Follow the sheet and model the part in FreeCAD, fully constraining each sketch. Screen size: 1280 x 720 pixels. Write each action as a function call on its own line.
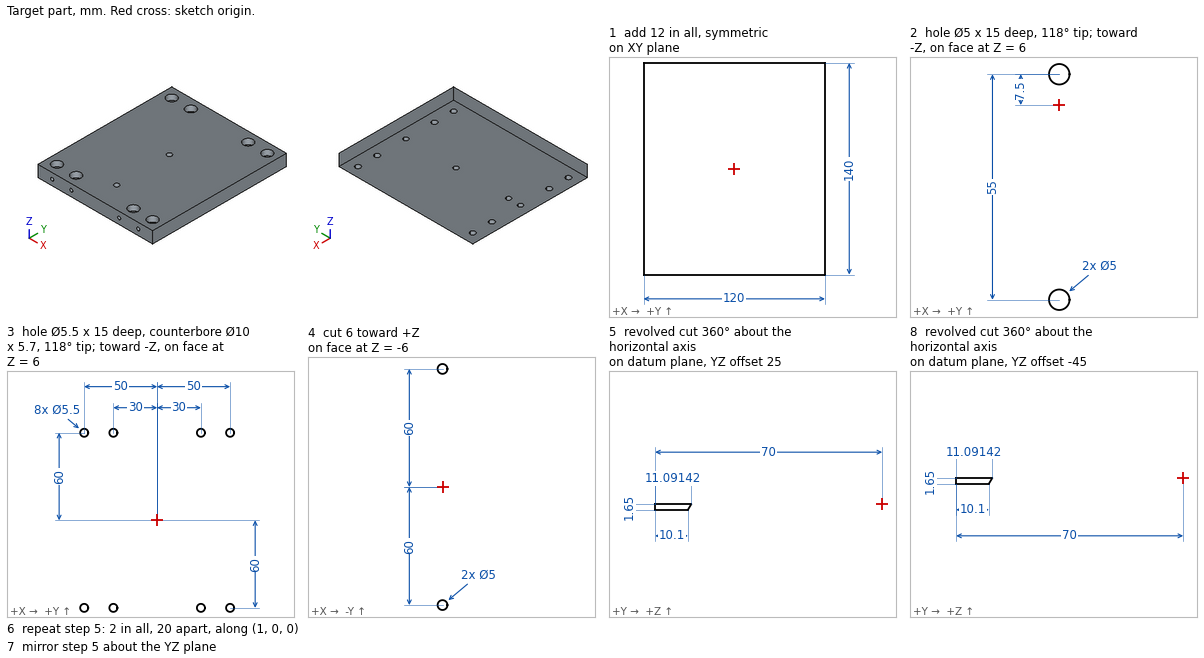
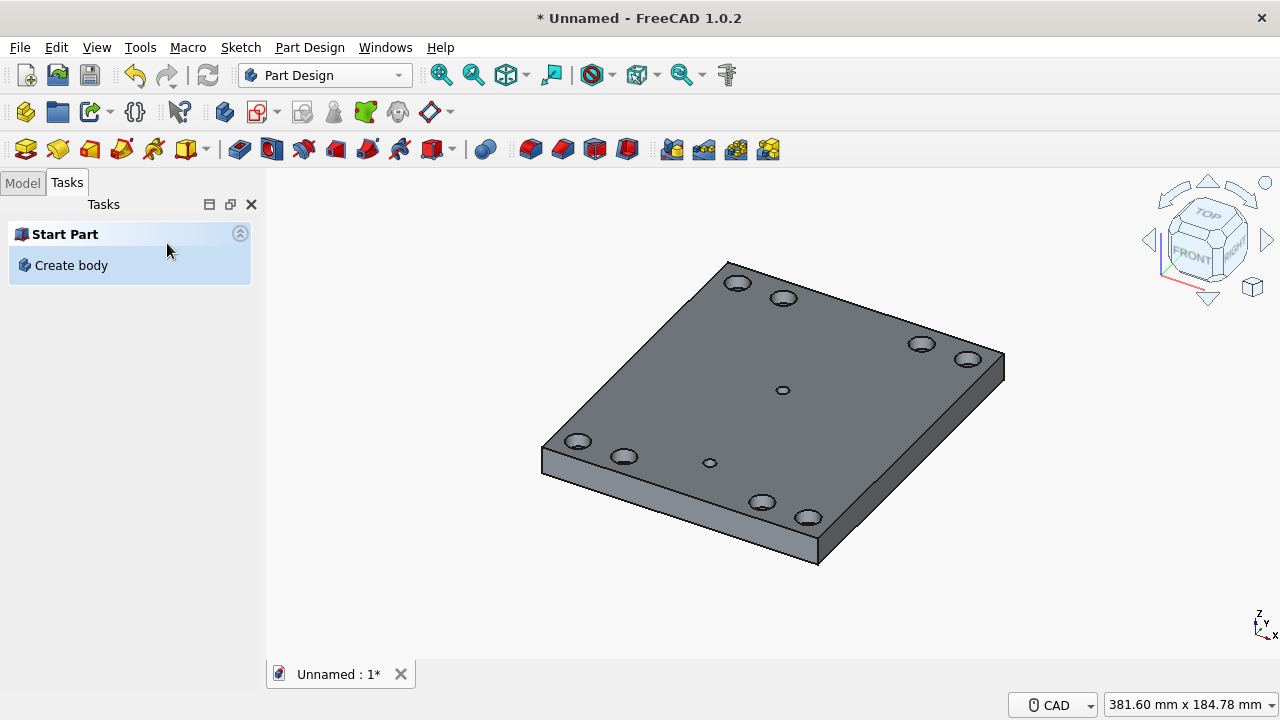
key(5)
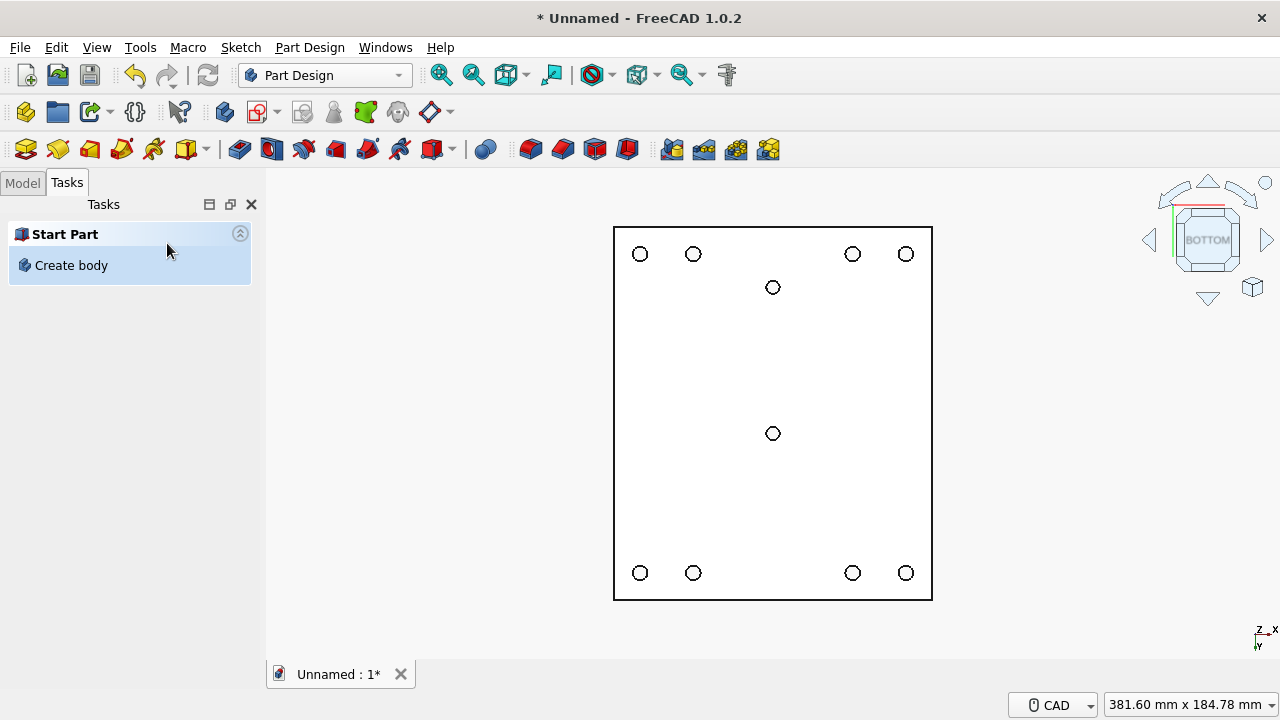
click(773, 519)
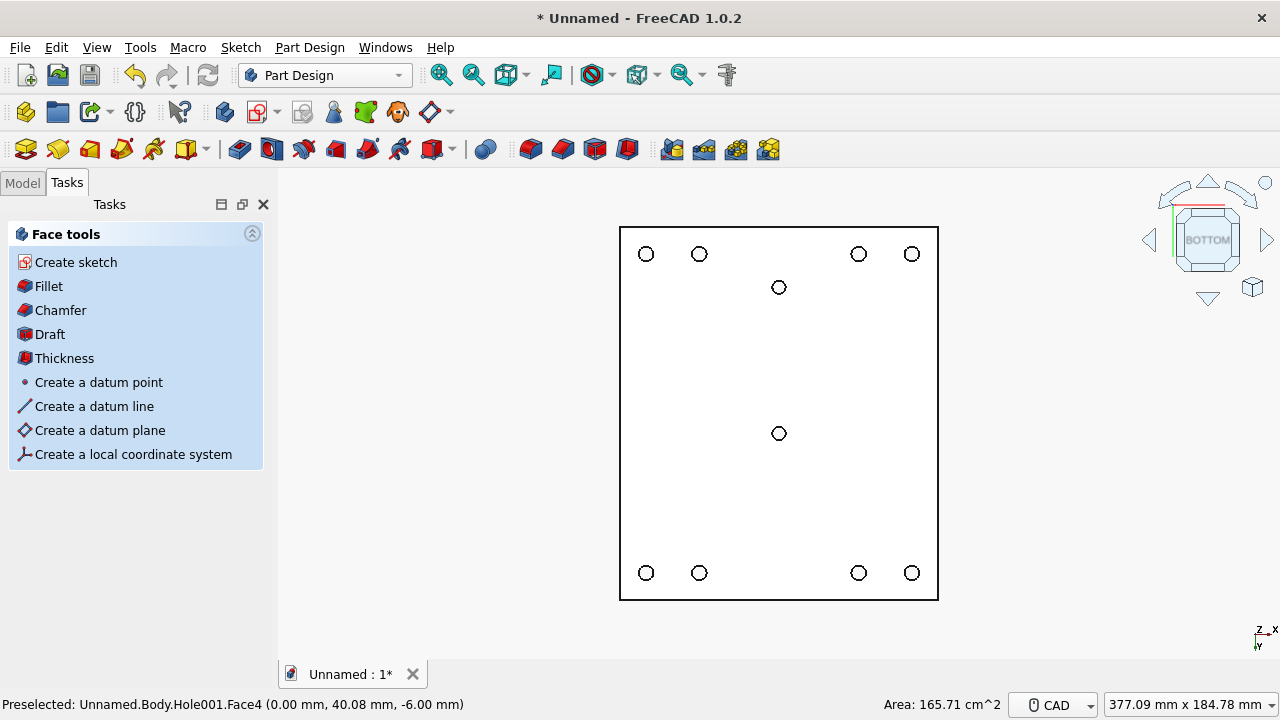
click(258, 112)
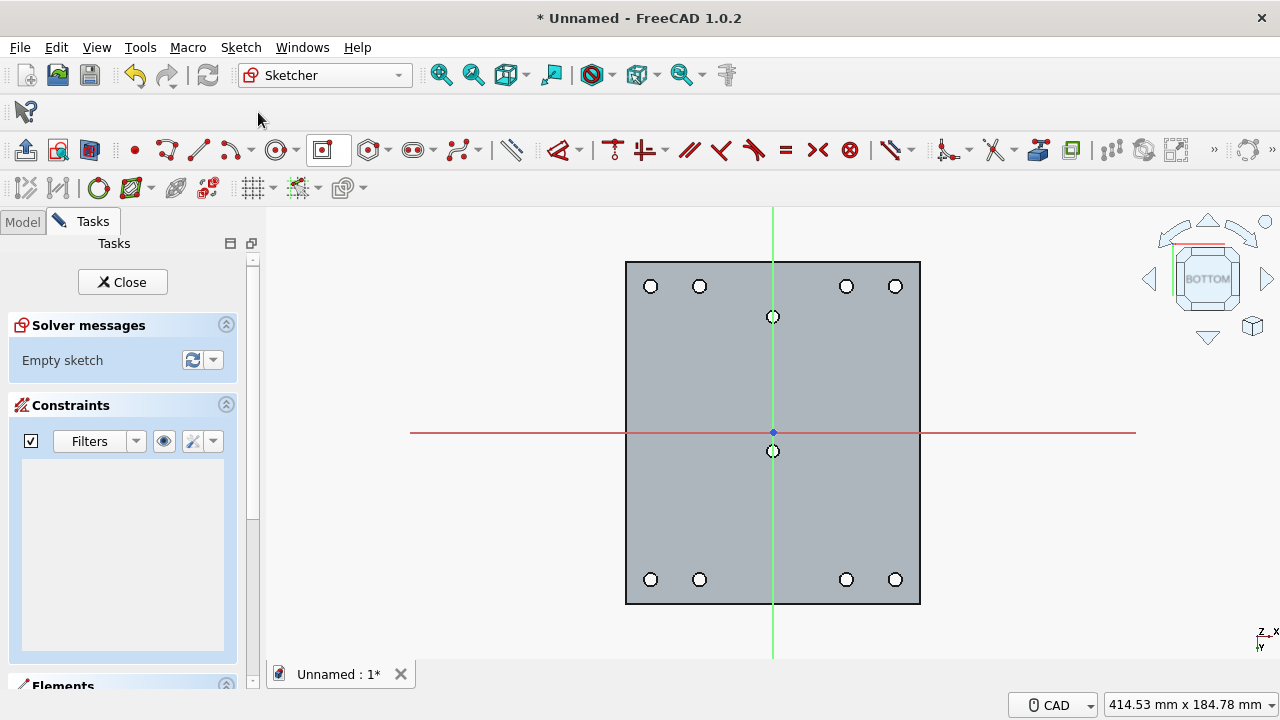
key(g)
key(c)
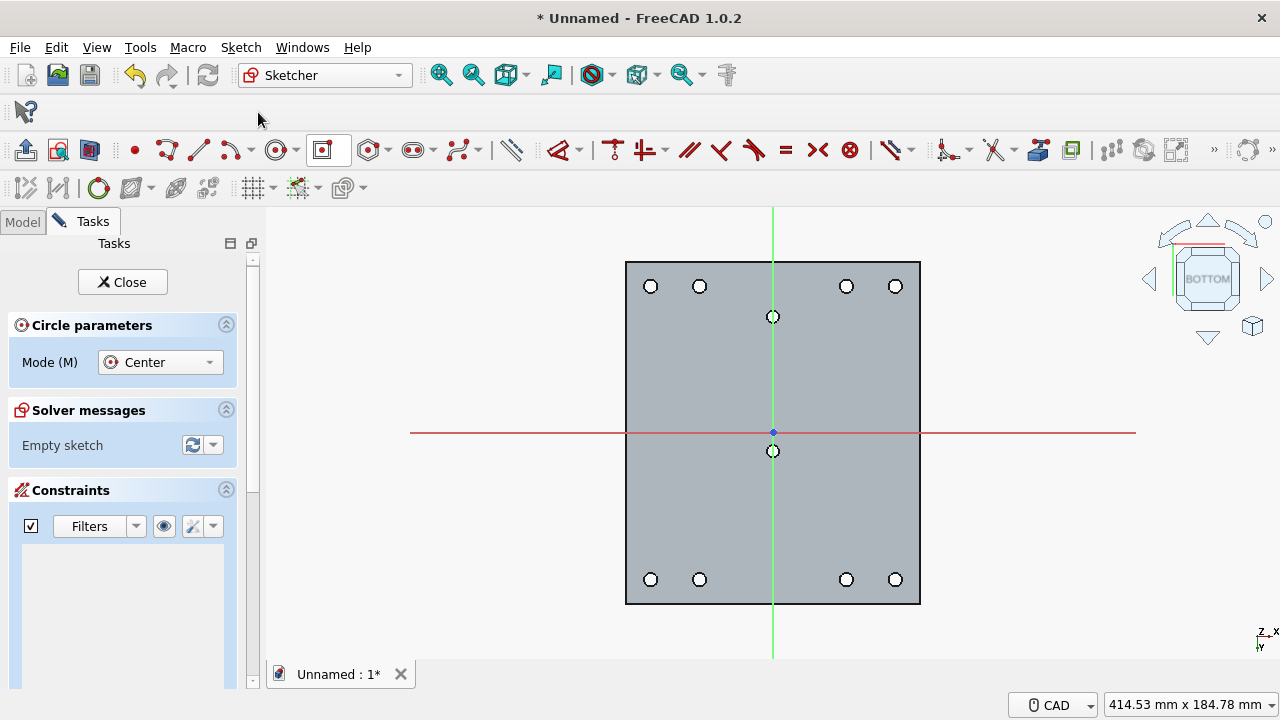
scroll(773, 580, up, 7)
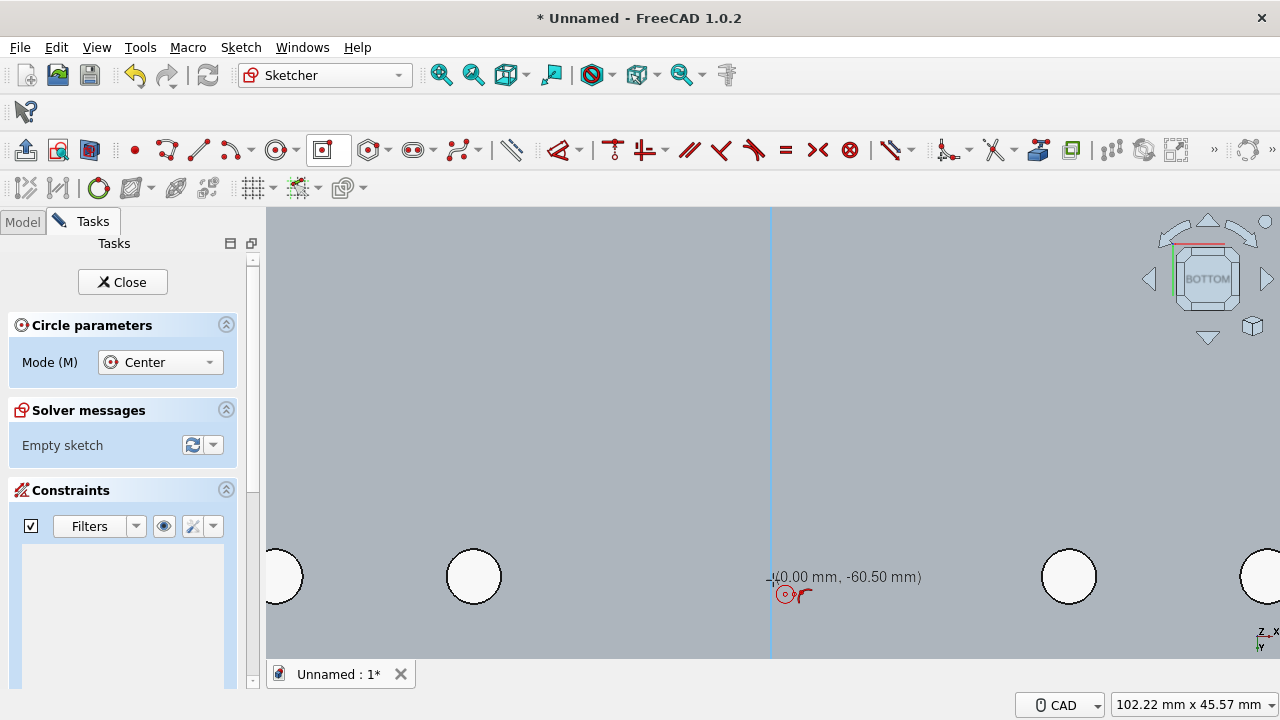
scroll(683, 581, down, 7)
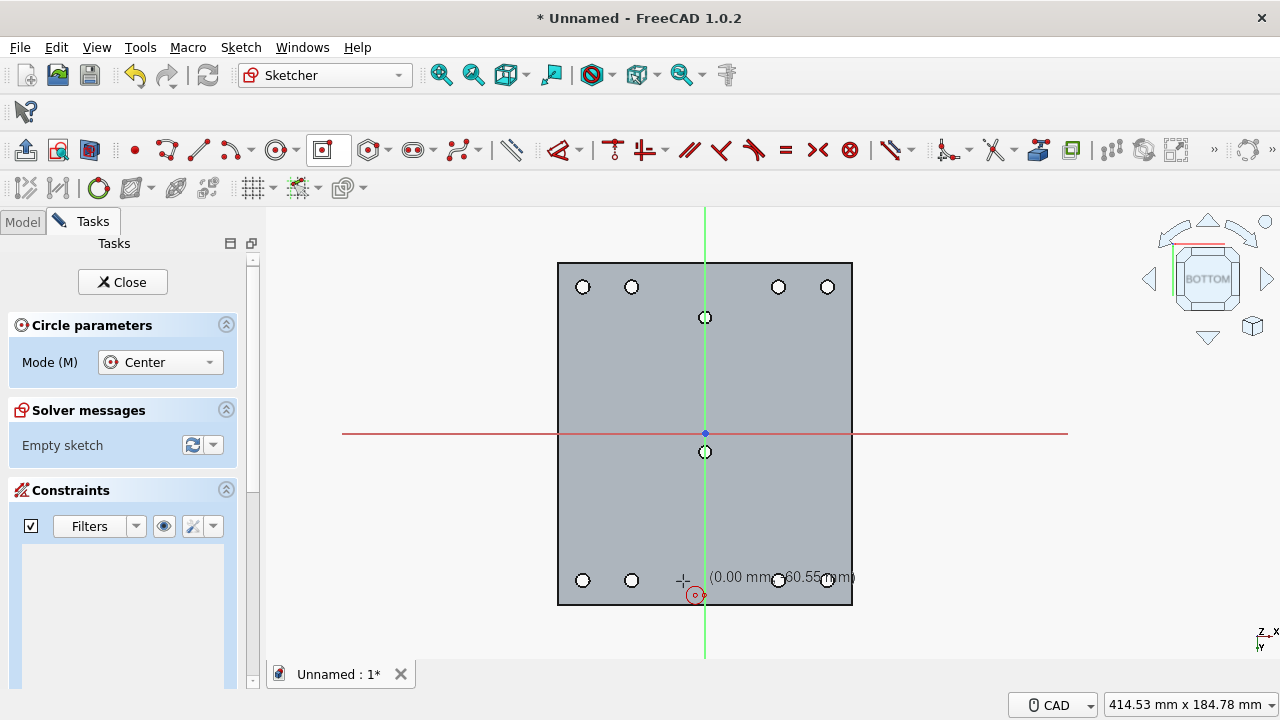
click(705, 581)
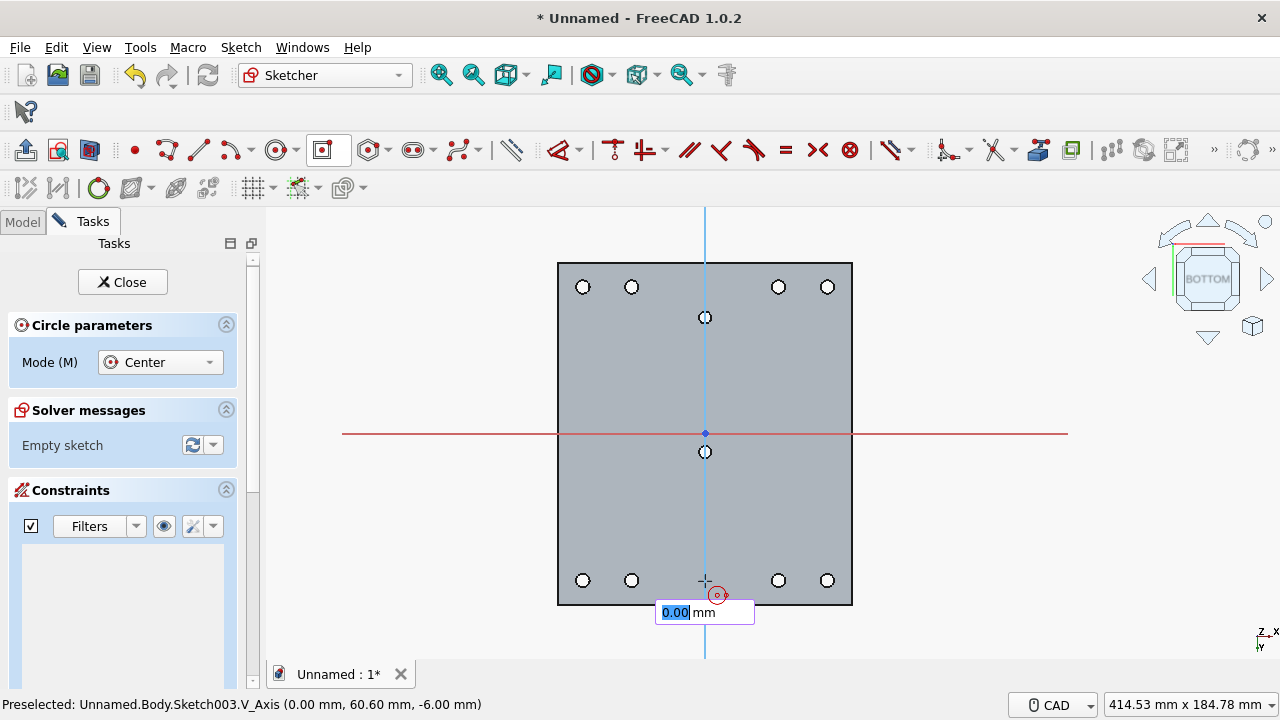
scroll(711, 578, up, 6)
move(710, 578)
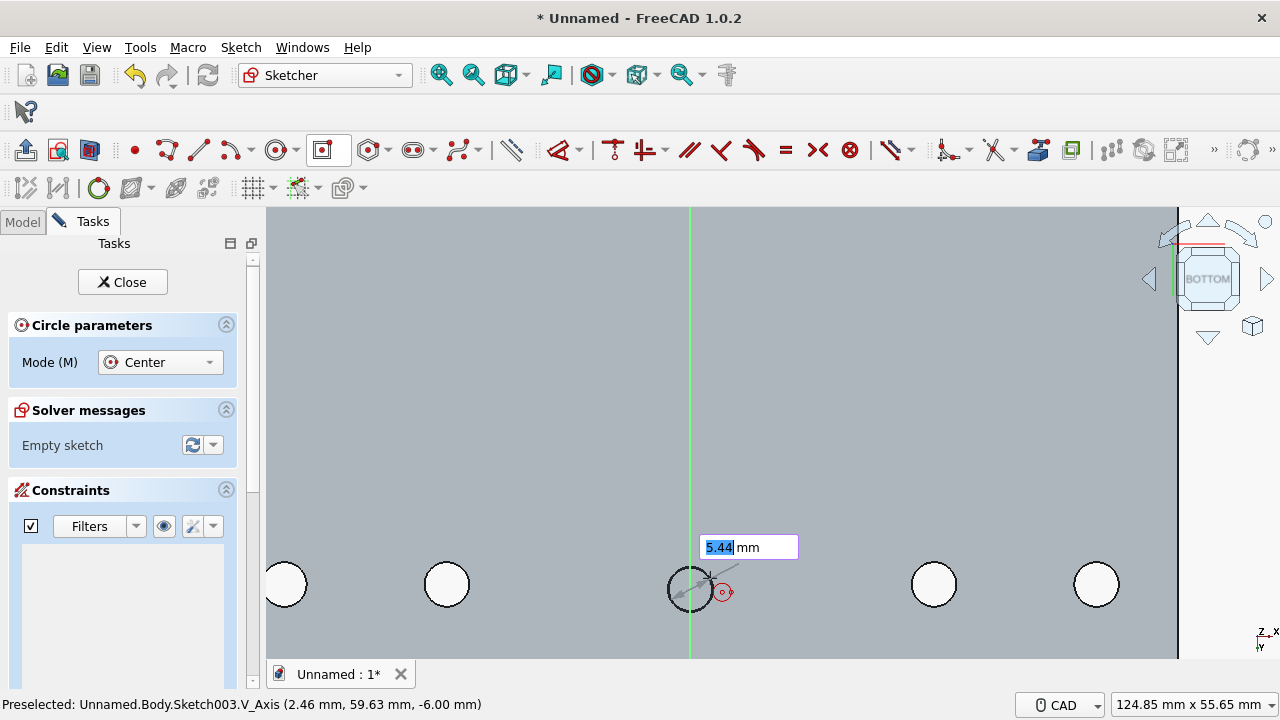
text(5)
key(Return)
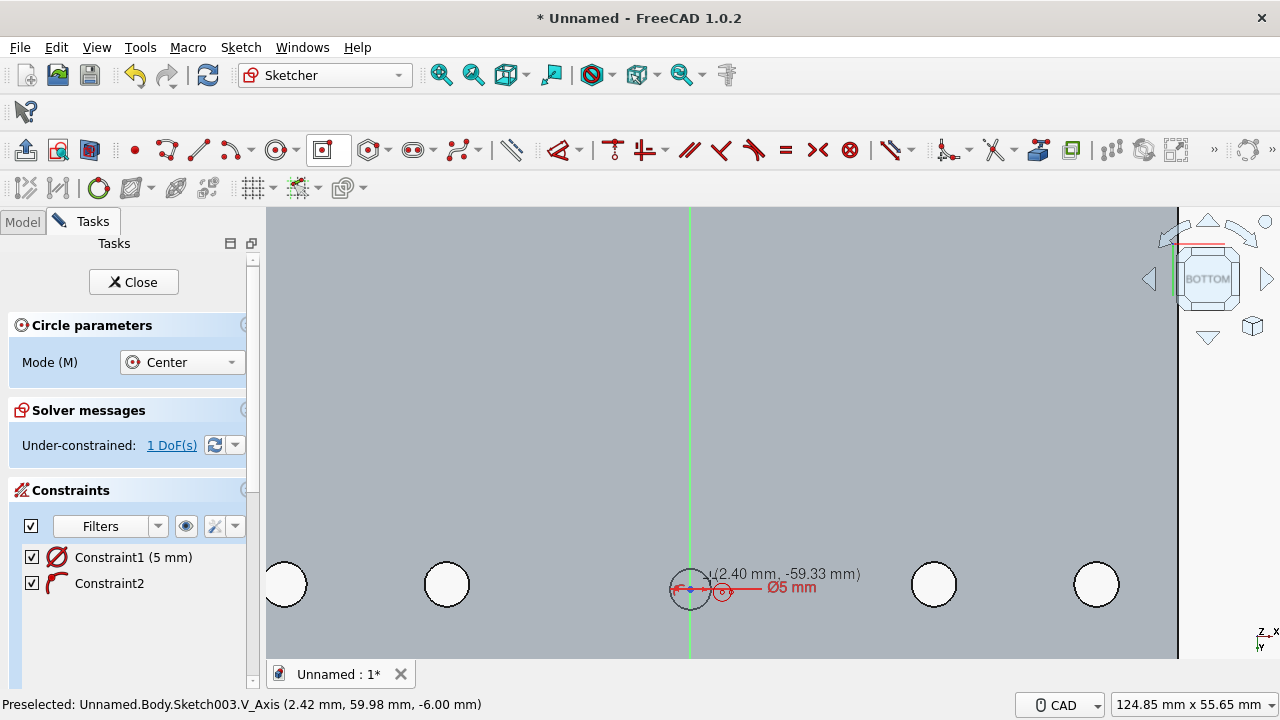
scroll(711, 578, down, 6)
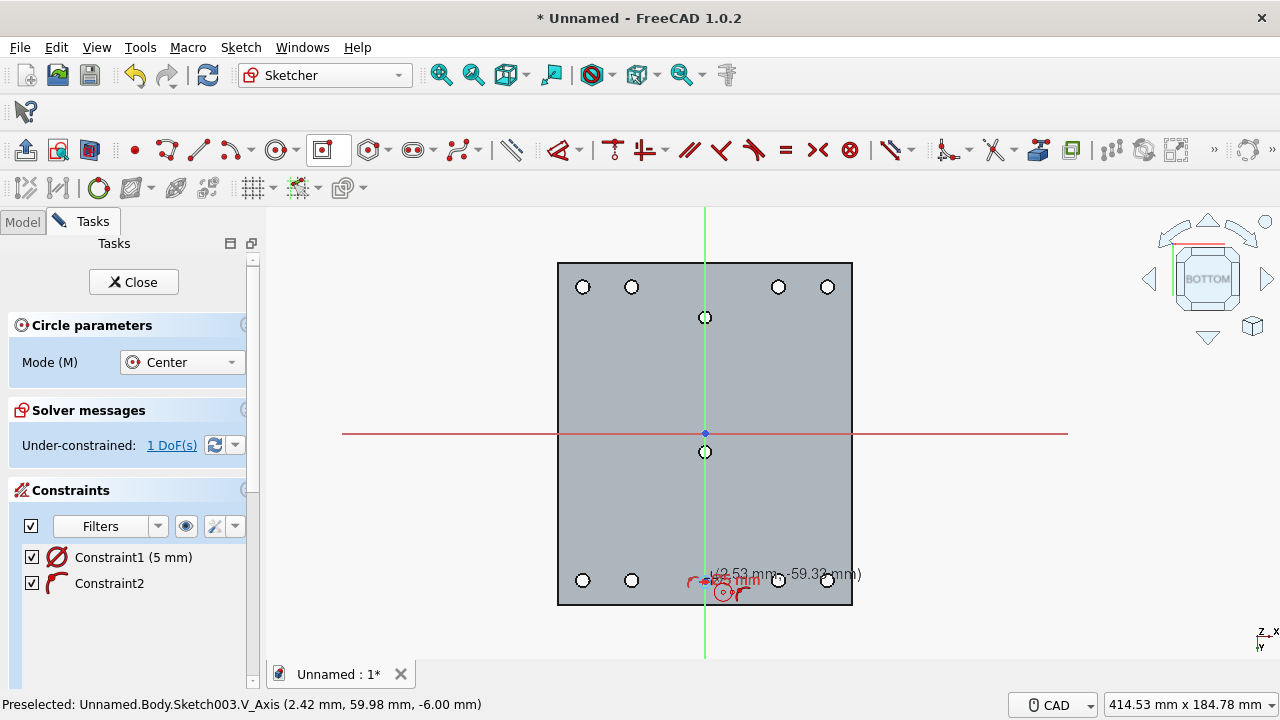
scroll(705, 287, up, 7)